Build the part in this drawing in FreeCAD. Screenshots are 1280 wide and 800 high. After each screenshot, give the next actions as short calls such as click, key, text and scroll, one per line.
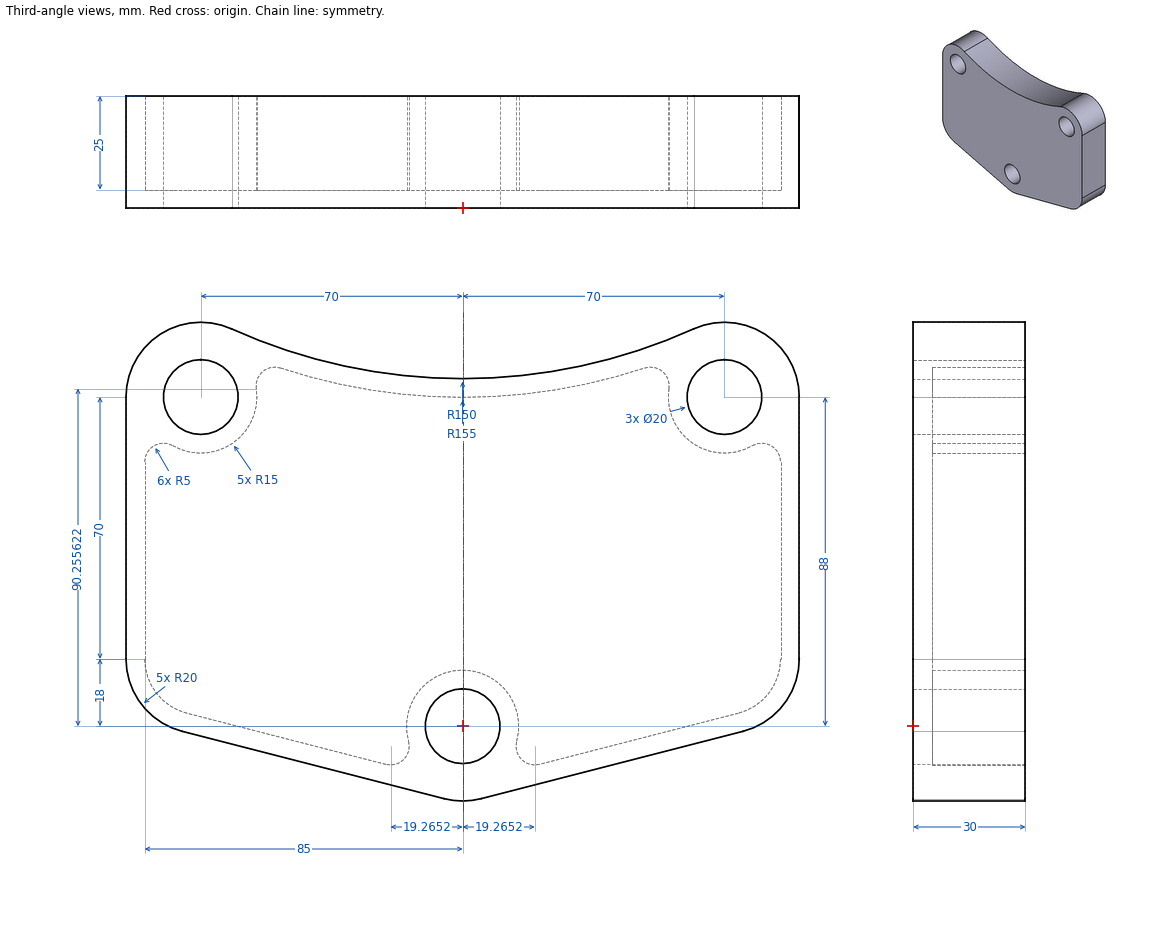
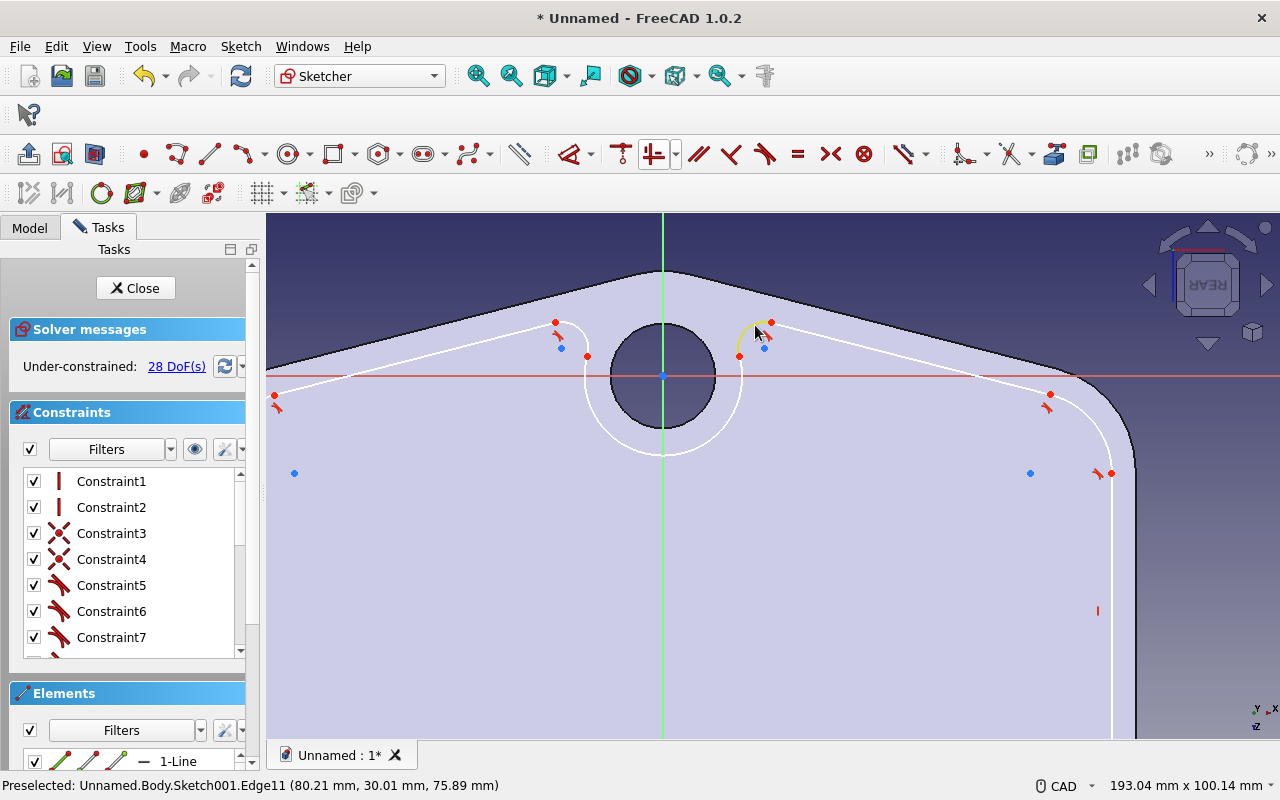
click(755, 324)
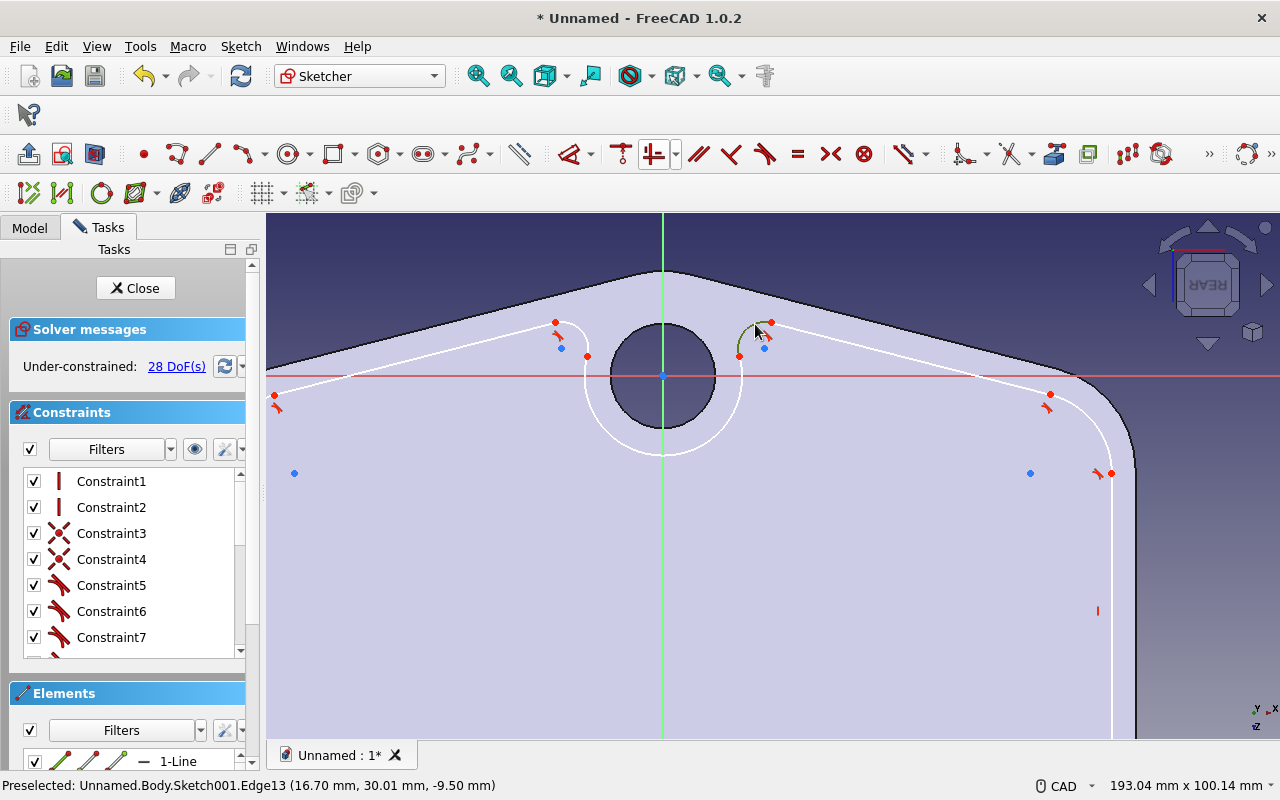
click(611, 435)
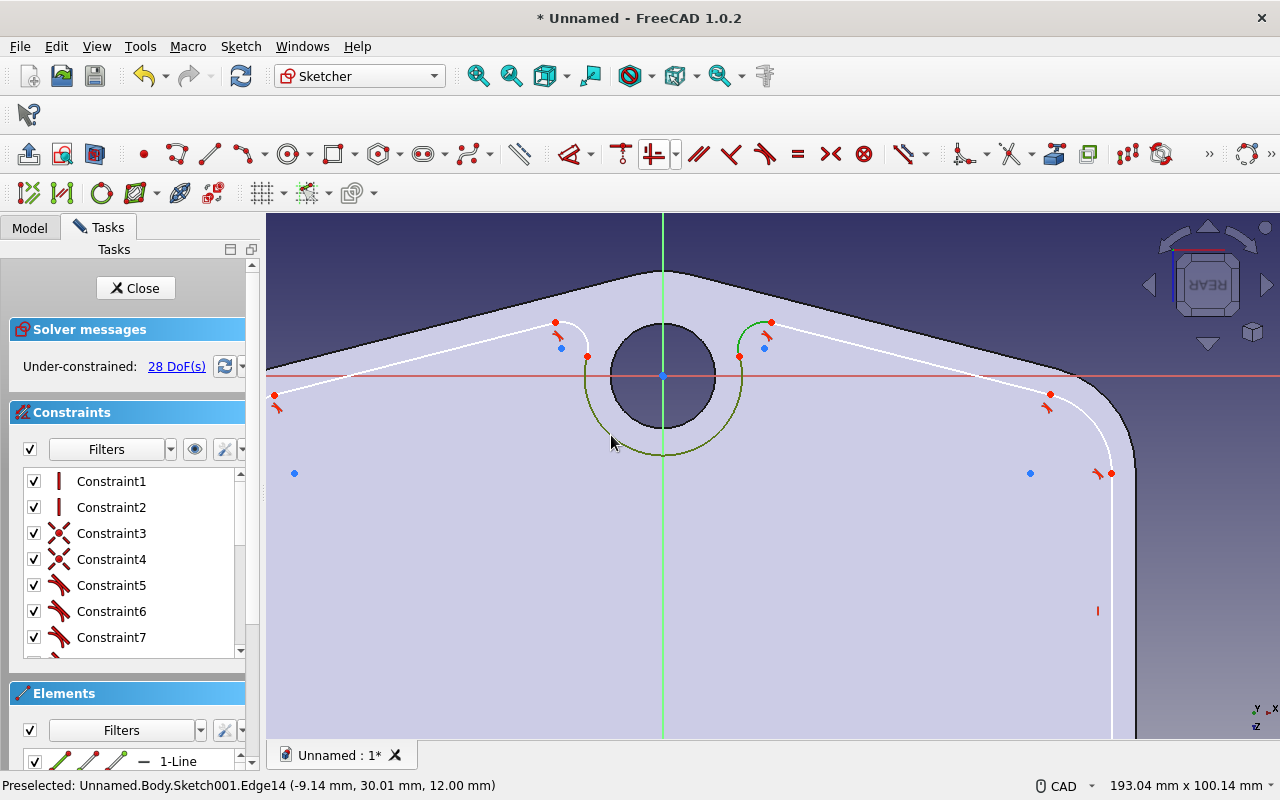
click(765, 154)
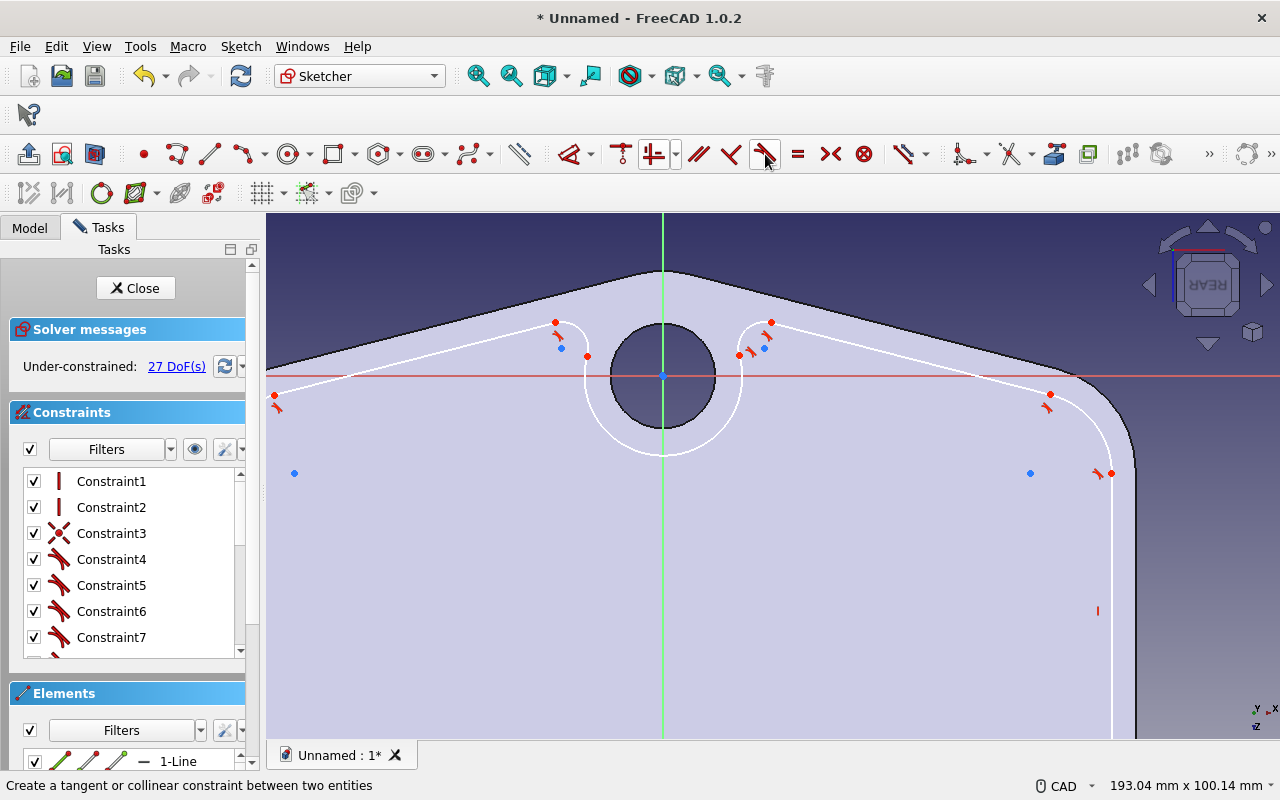
click(611, 435)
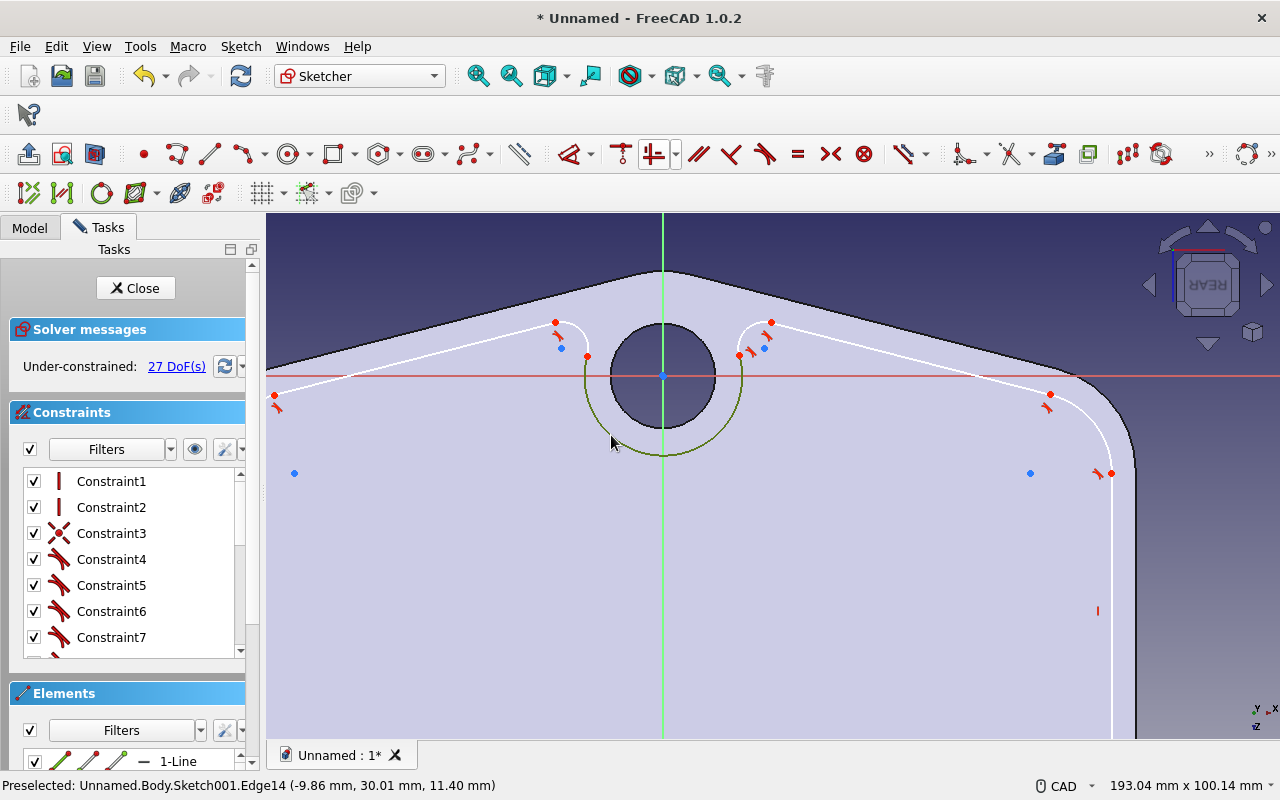
click(587, 340)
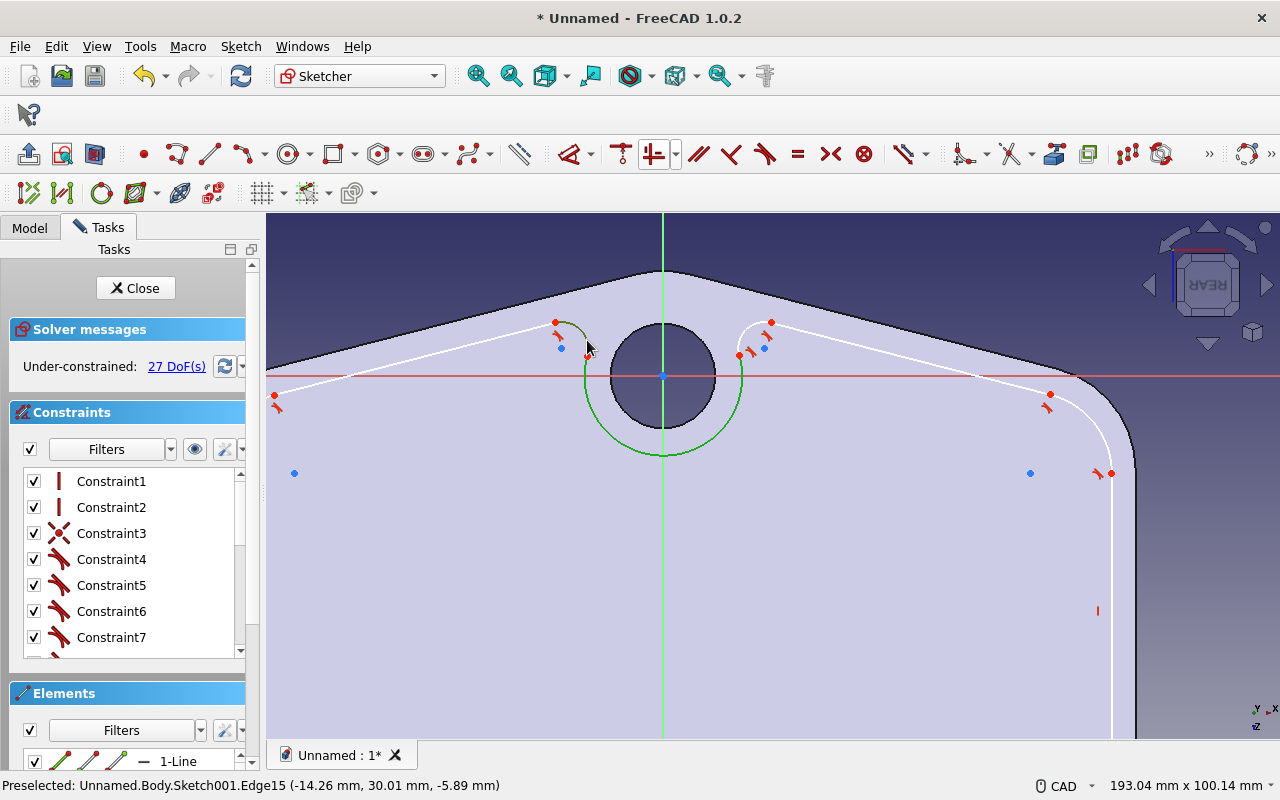
click(765, 154)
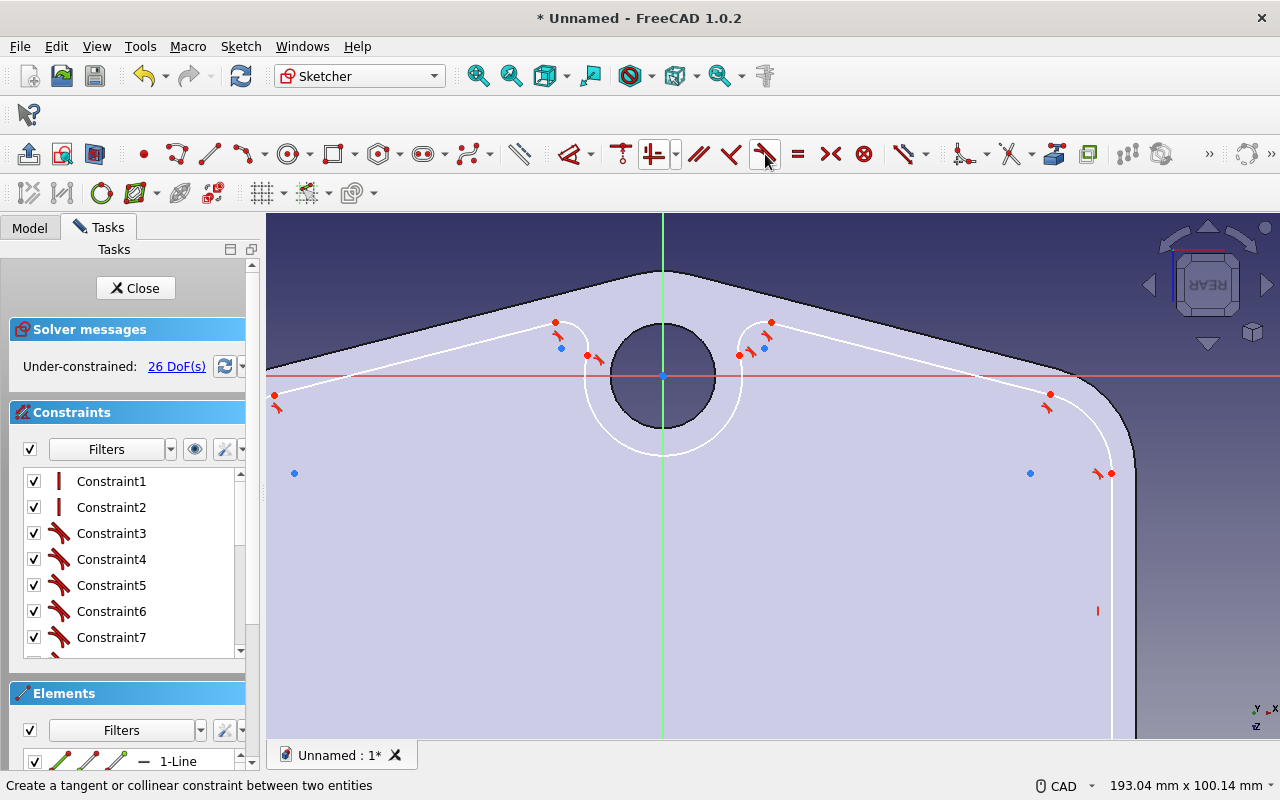
scroll(663, 376, up, 3)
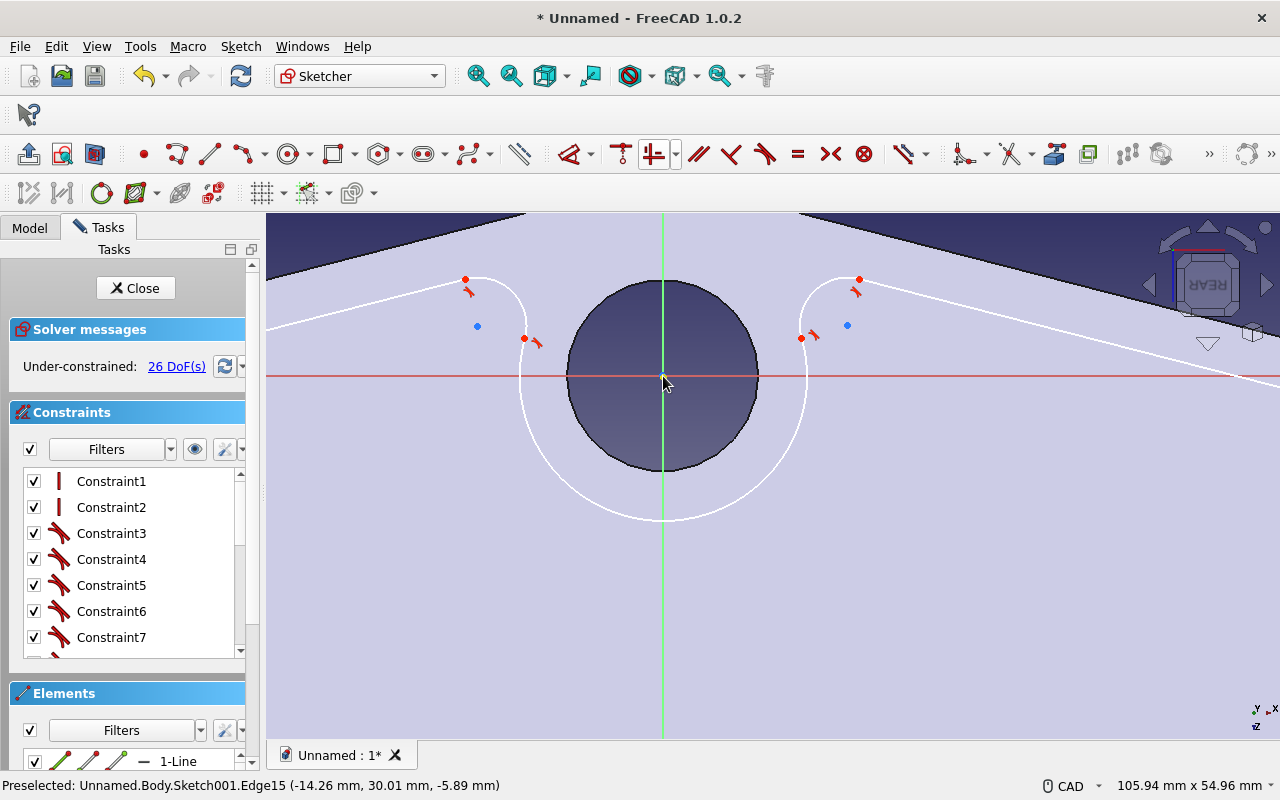
drag(653, 366, 673, 387)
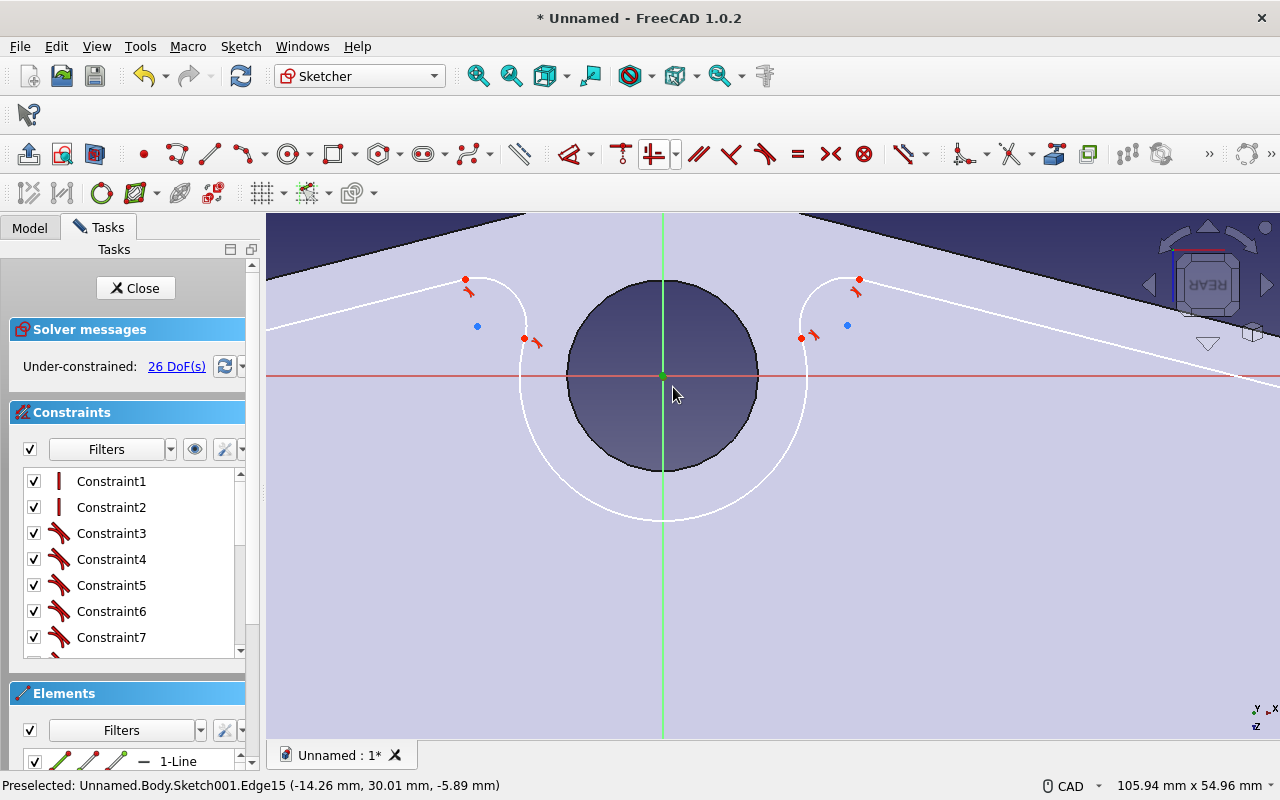
click(621, 154)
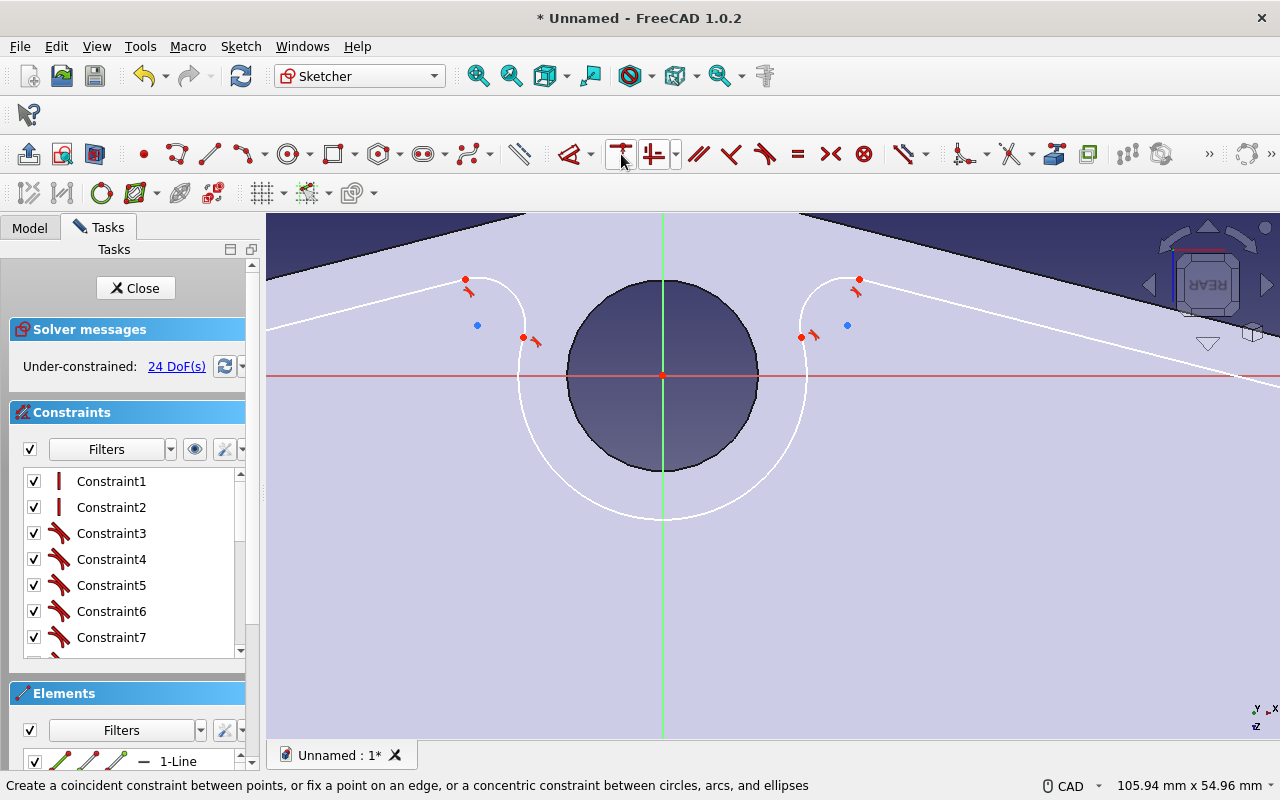
scroll(723, 343, down, 6)